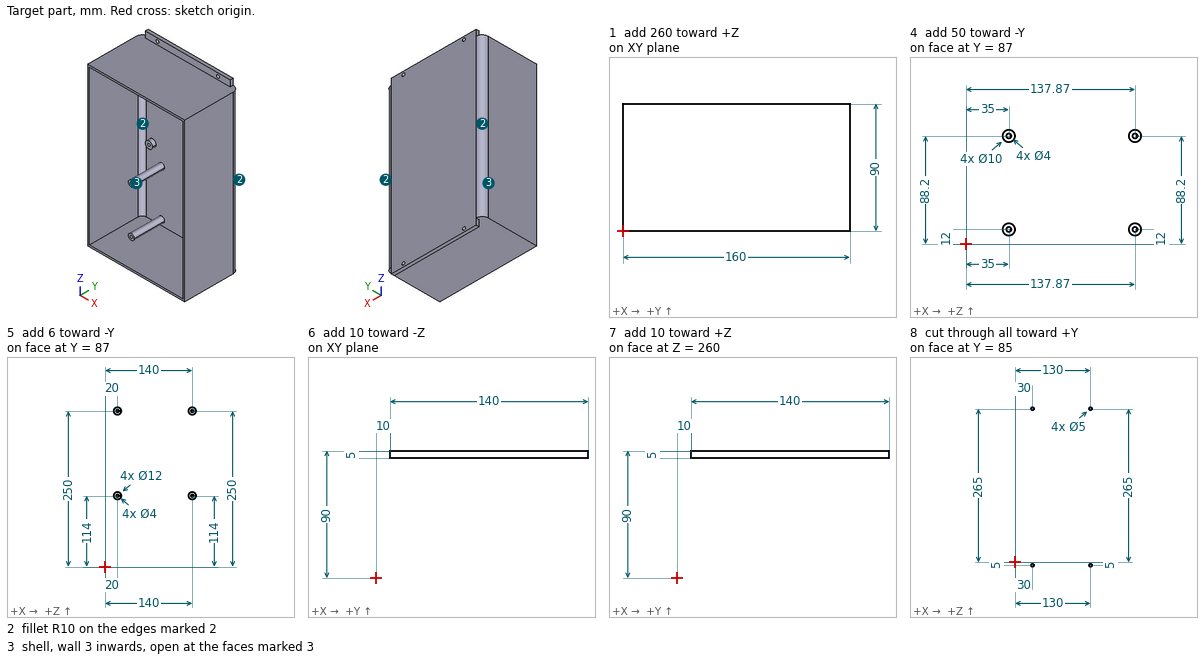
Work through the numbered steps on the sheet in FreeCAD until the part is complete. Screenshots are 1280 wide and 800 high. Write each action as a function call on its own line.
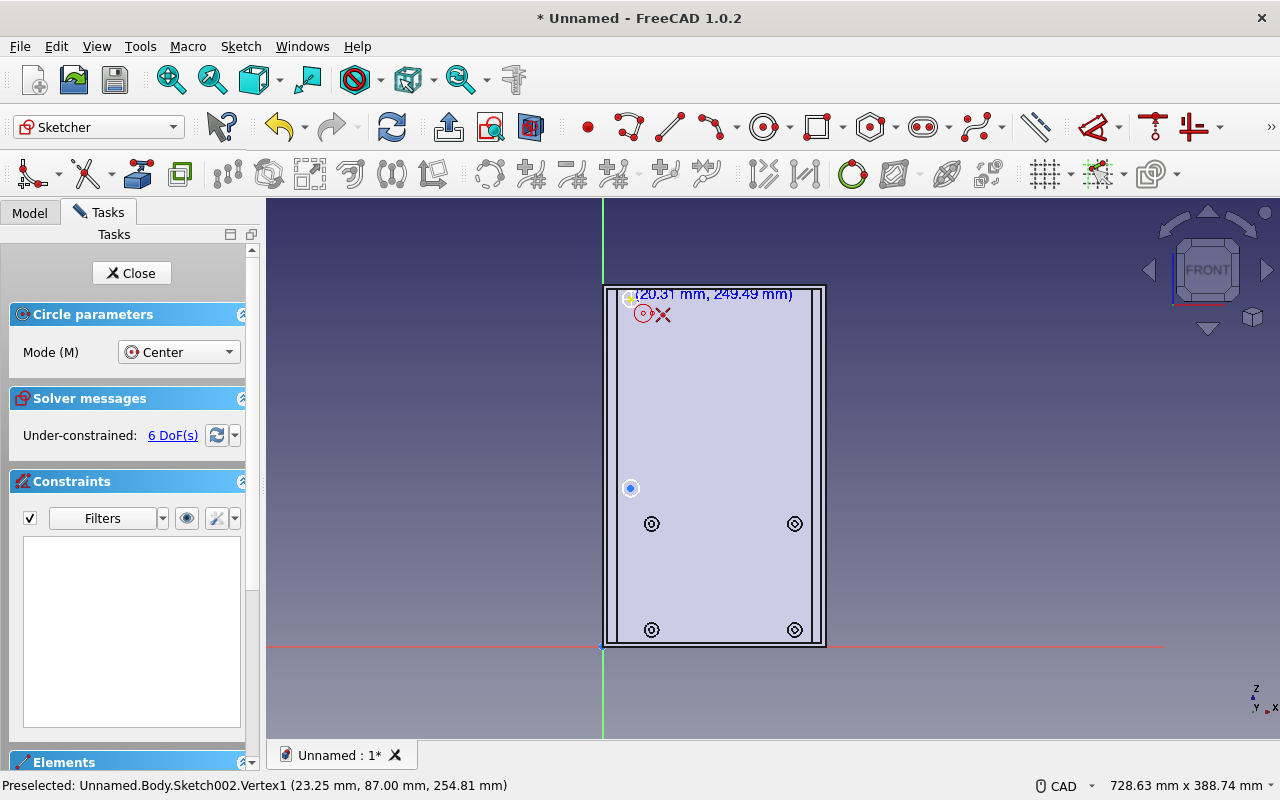
scroll(798, 488, up, 5)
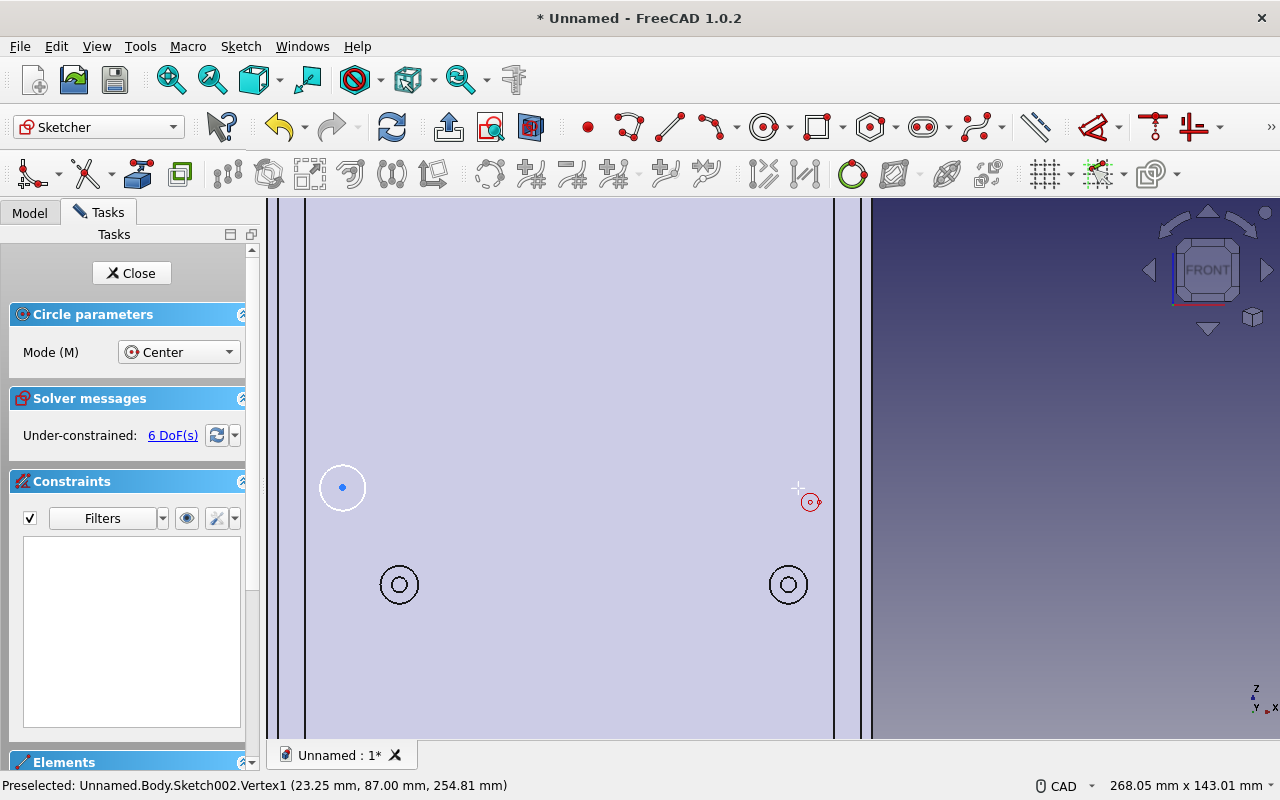
click(797, 487)
click(813, 471)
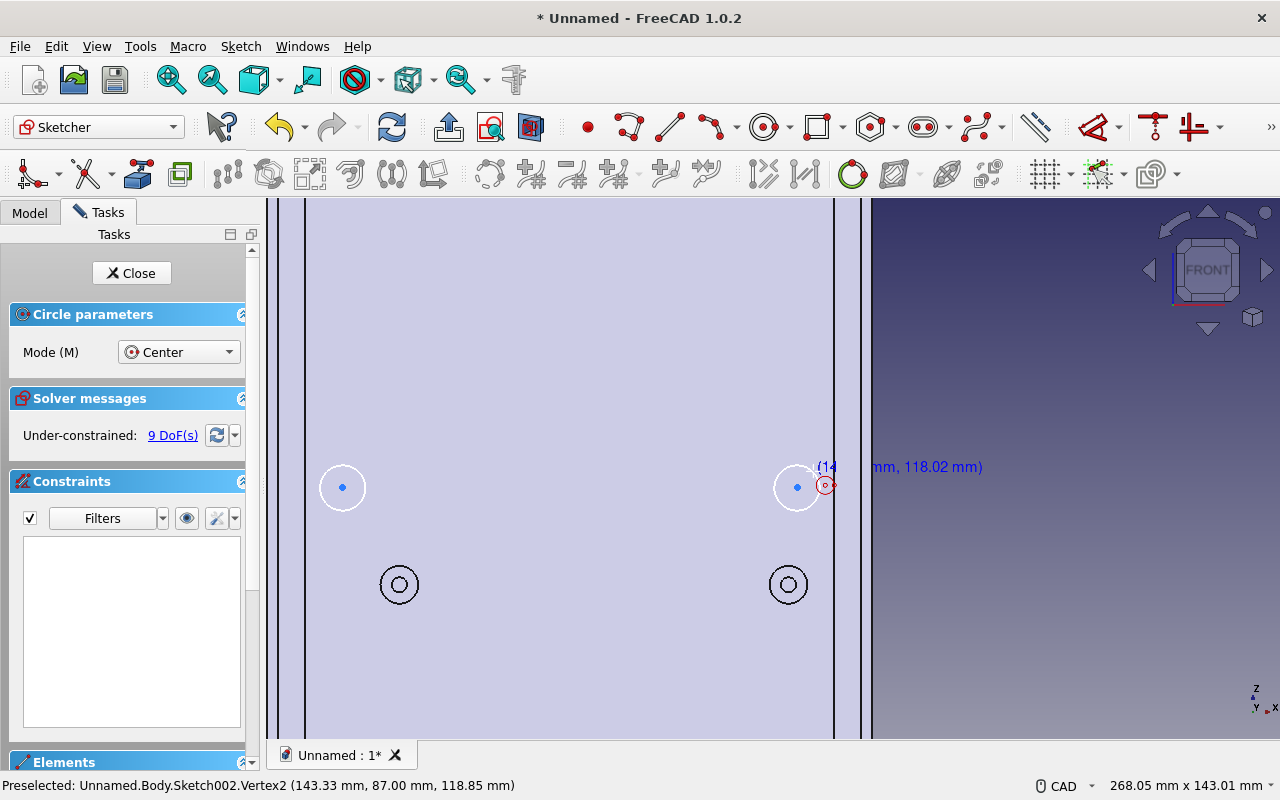
scroll(798, 488, down, 5)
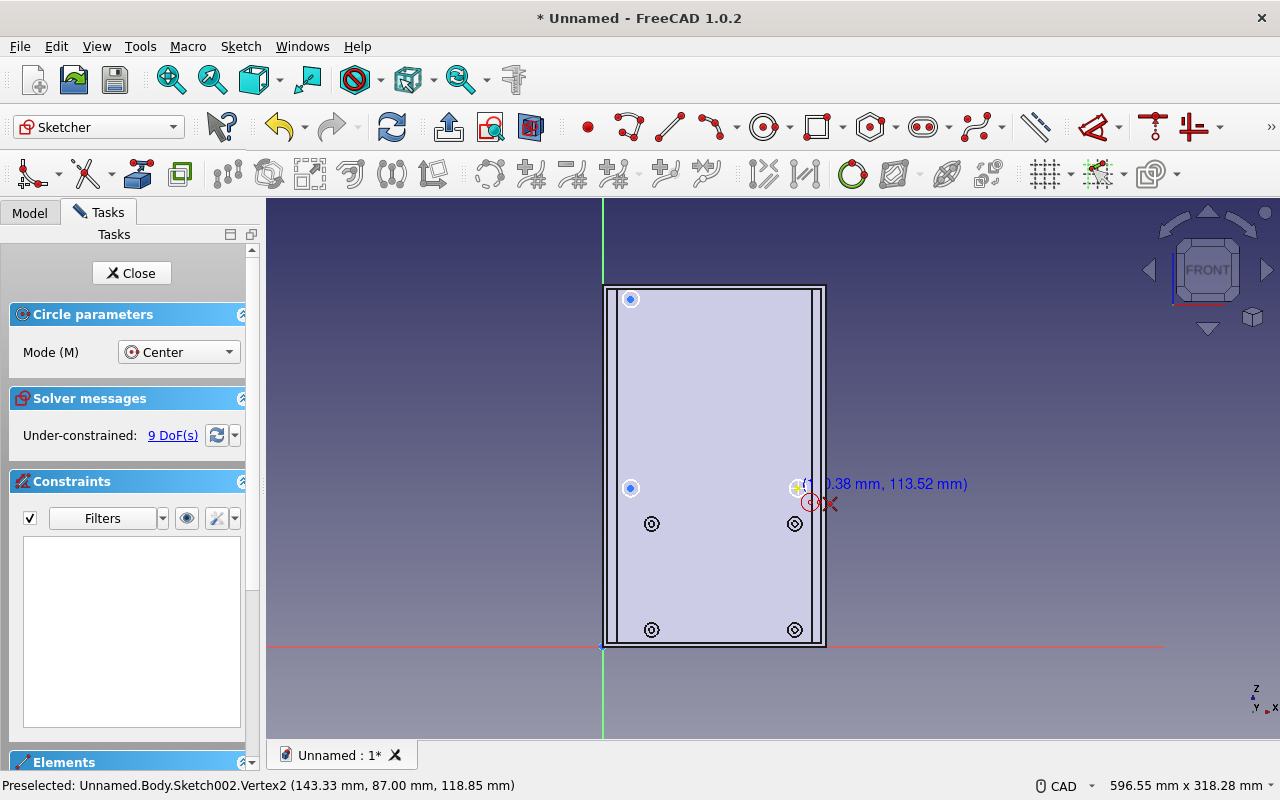
scroll(798, 299, up, 5)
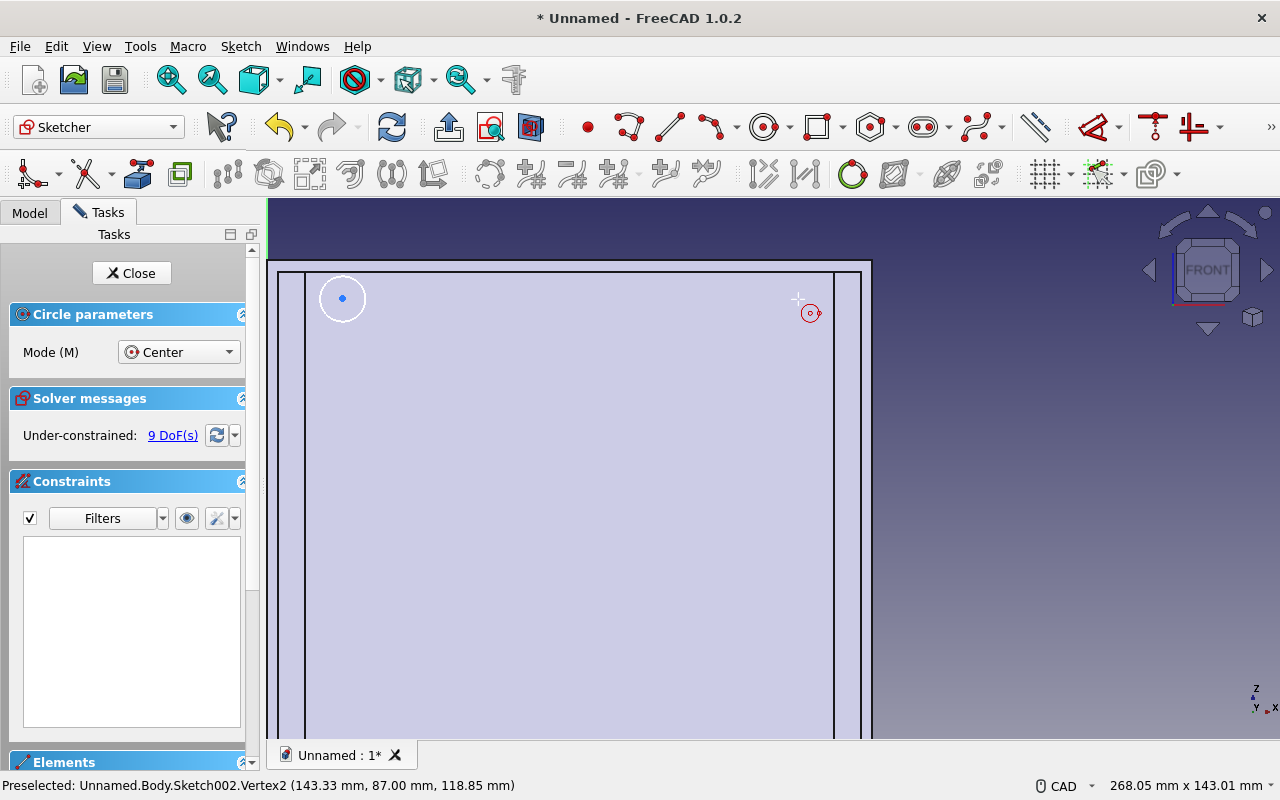
click(797, 298)
click(813, 282)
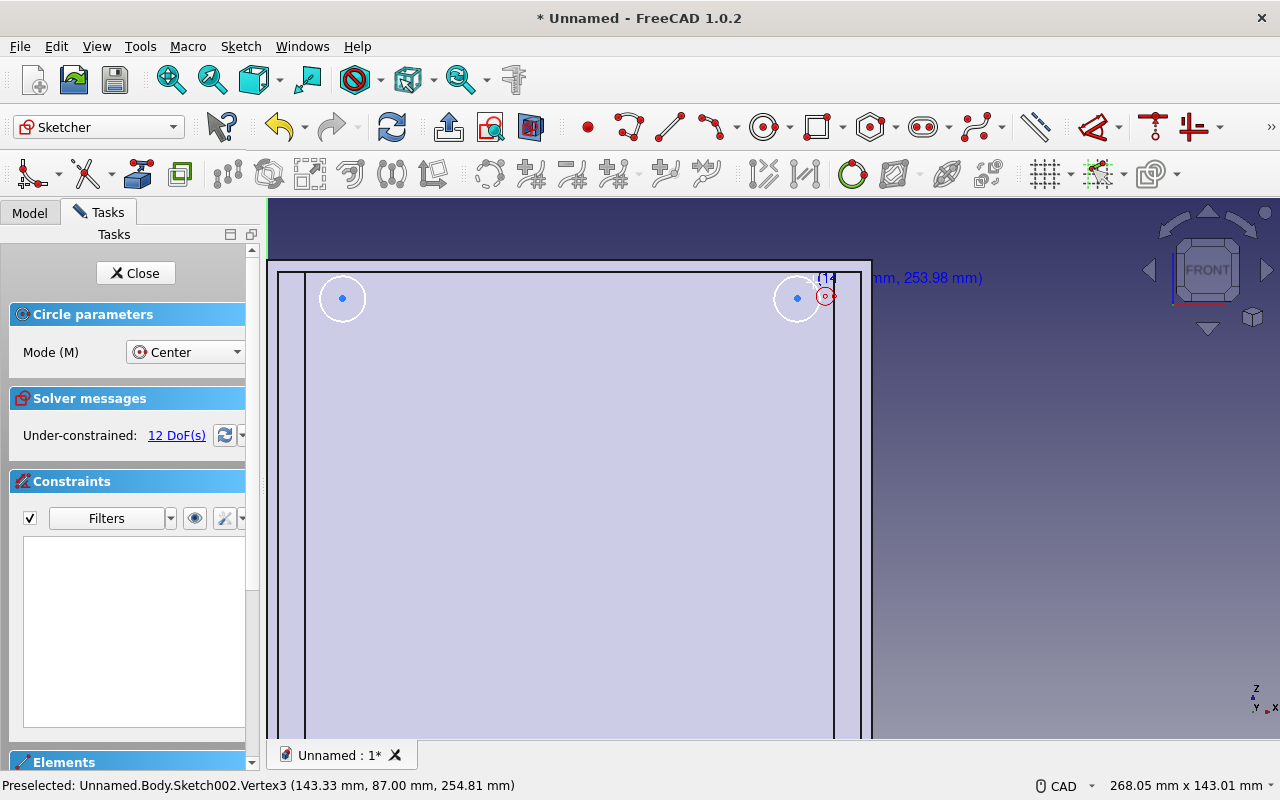
scroll(798, 299, down, 5)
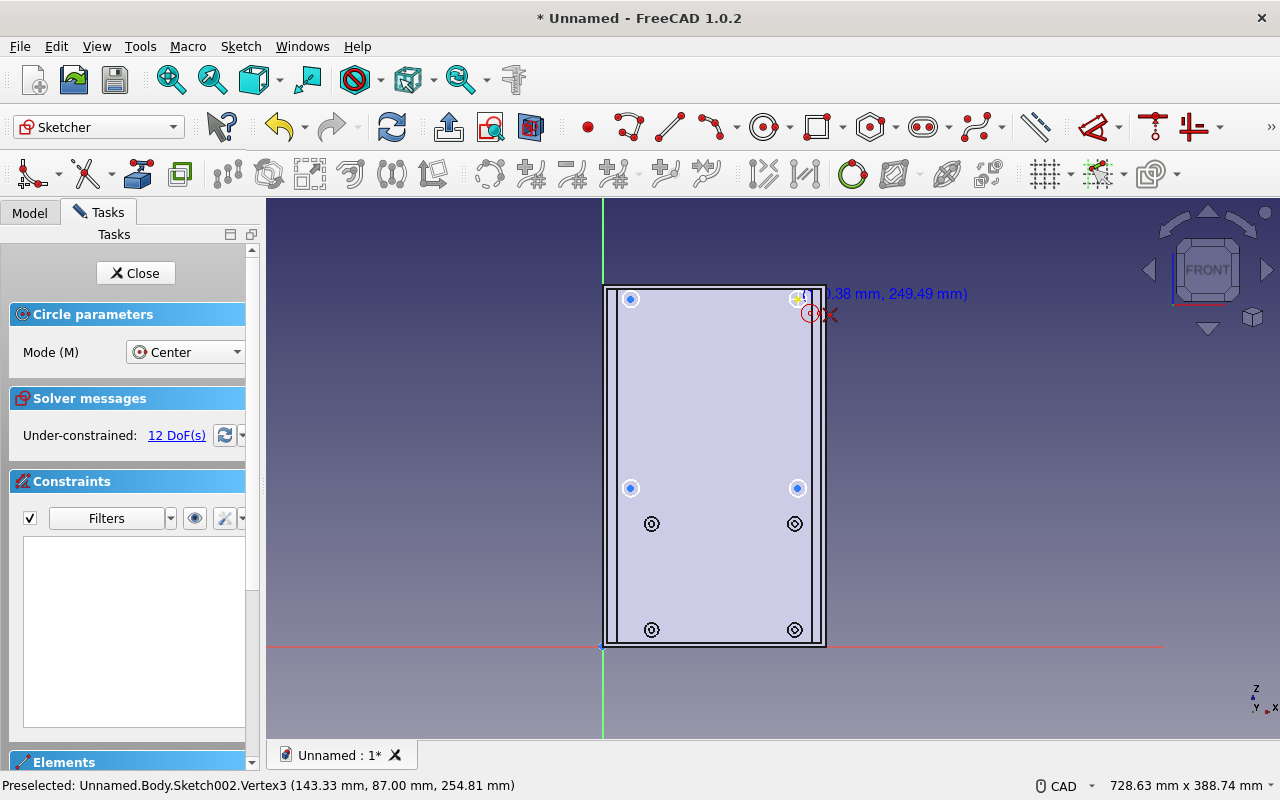
scroll(631, 488, up, 11)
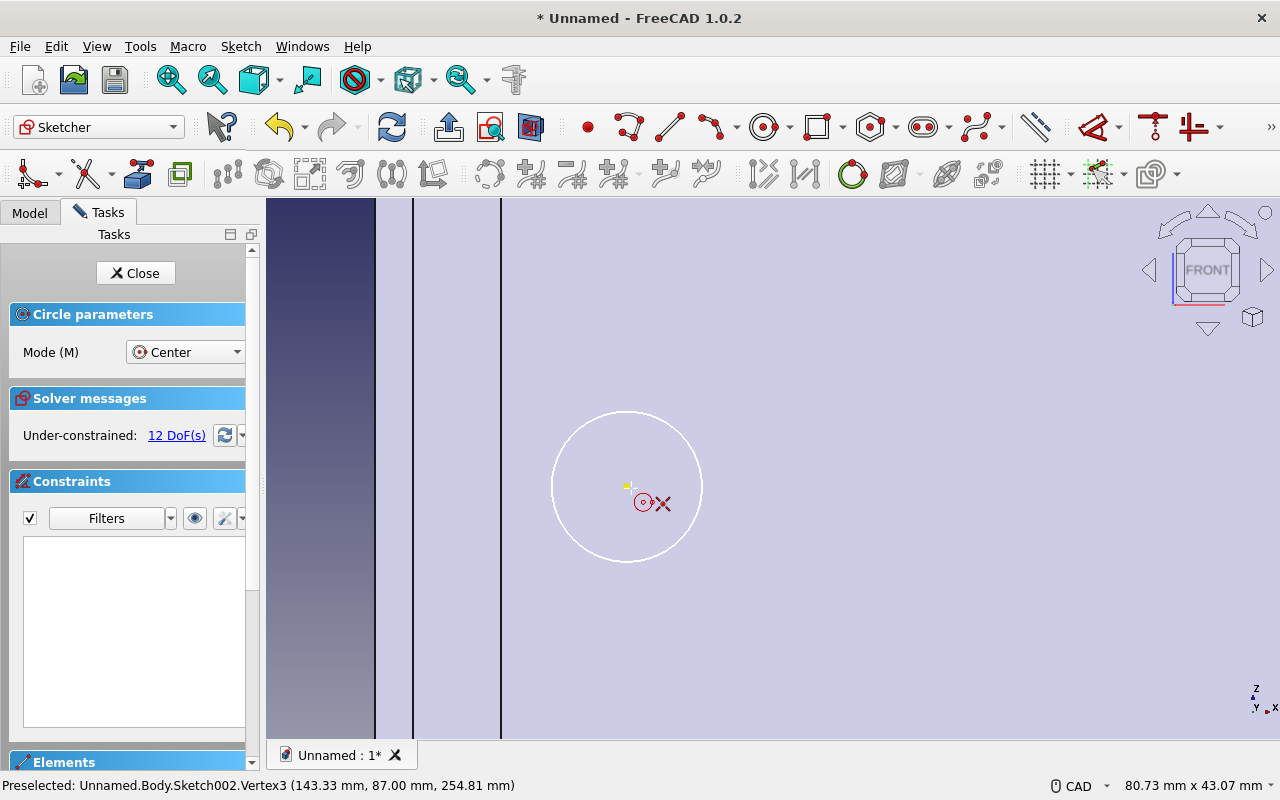
scroll(631, 488, down, 11)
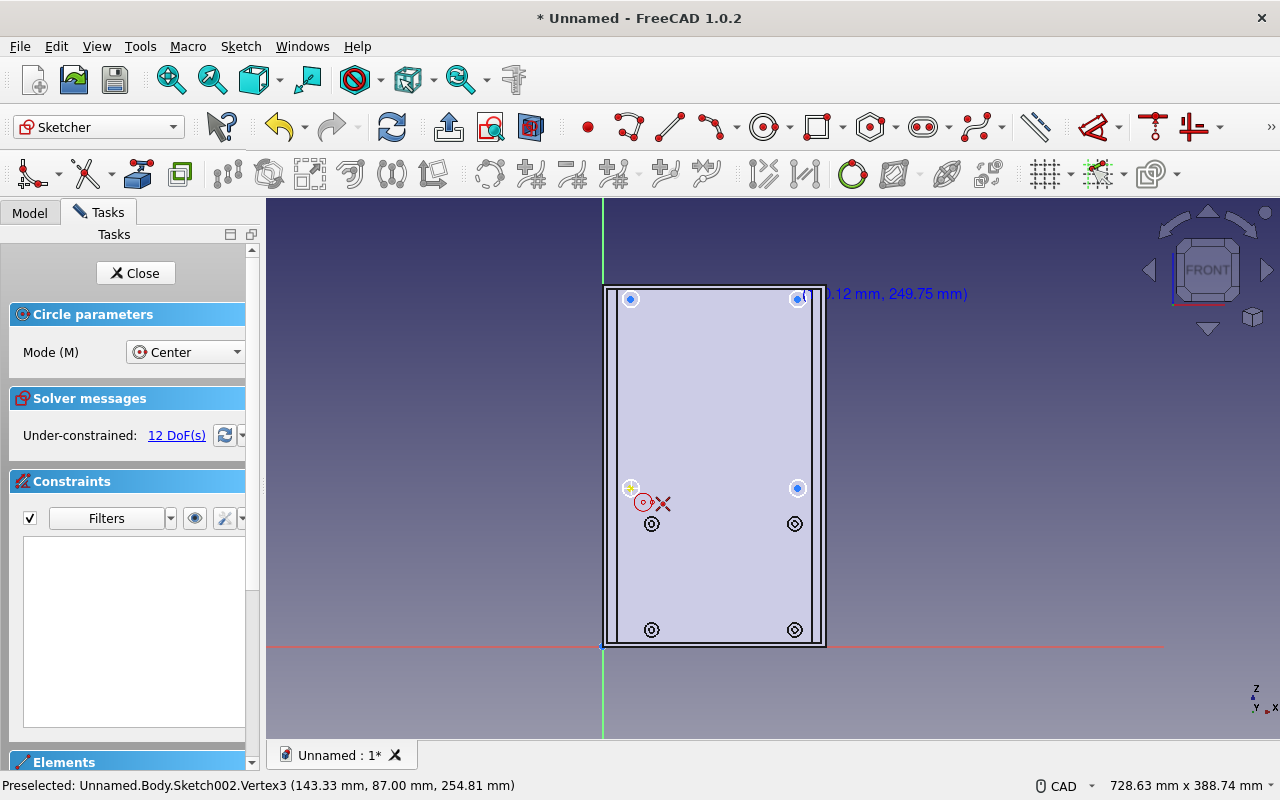
scroll(631, 488, up, 4)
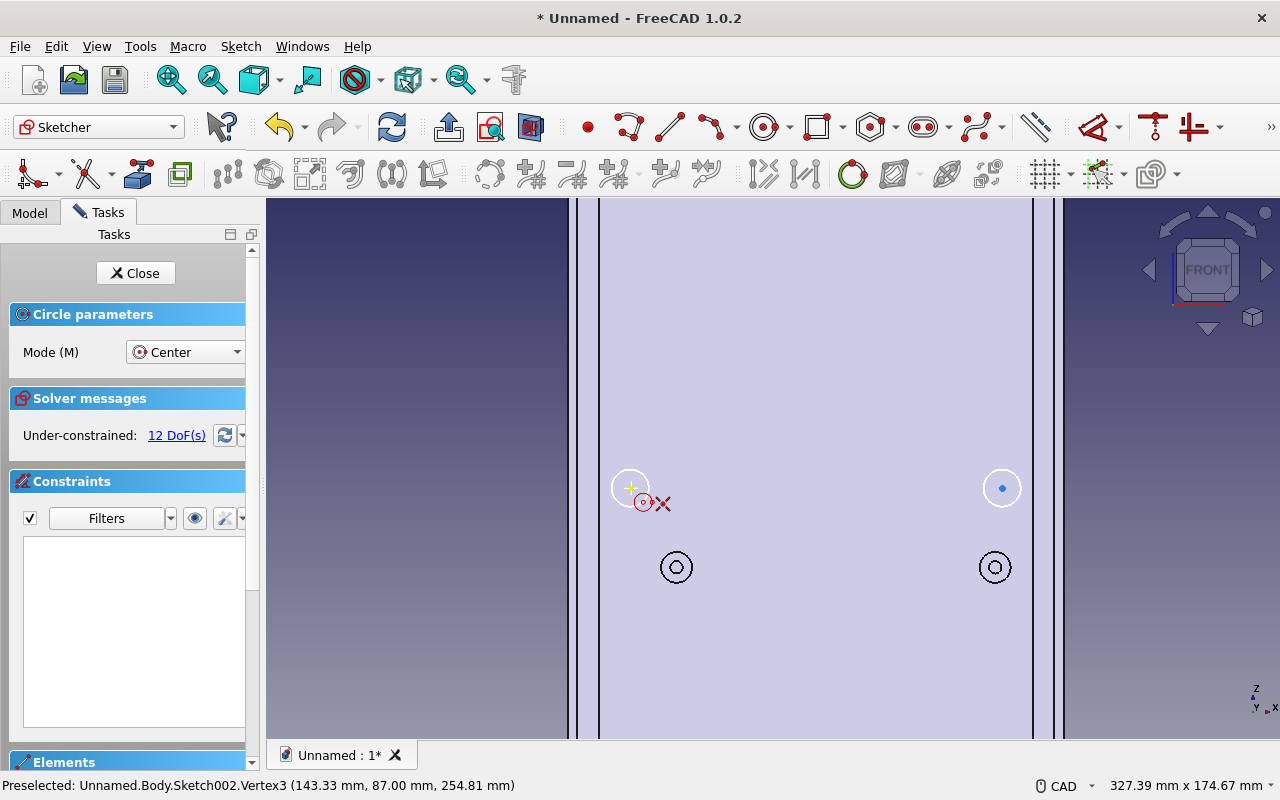
click(630, 488)